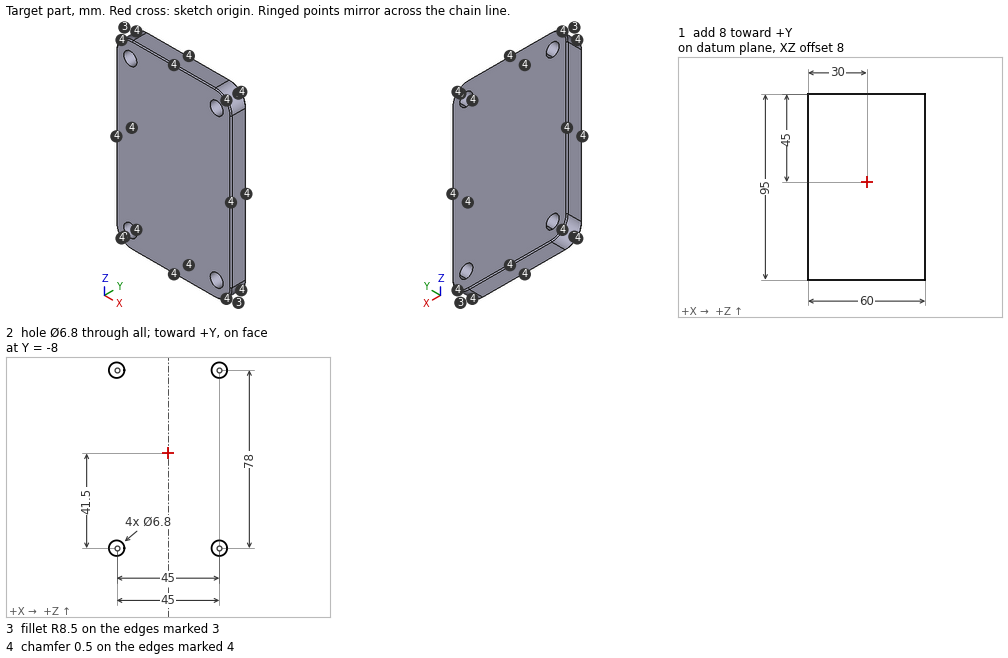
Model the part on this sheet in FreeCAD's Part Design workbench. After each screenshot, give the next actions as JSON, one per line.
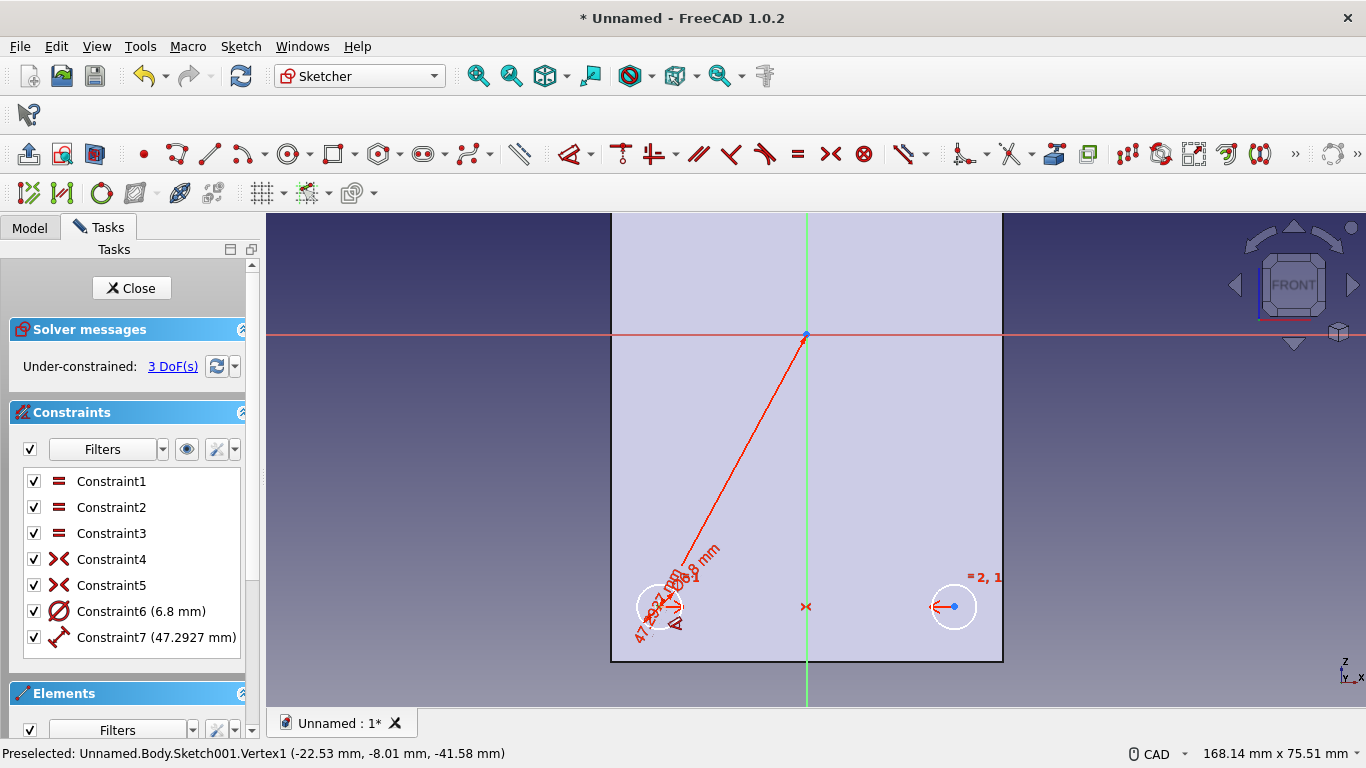
{"action": "left_click", "coordinate": [954, 607]}
{"action": "left_click", "coordinate": [739, 641]}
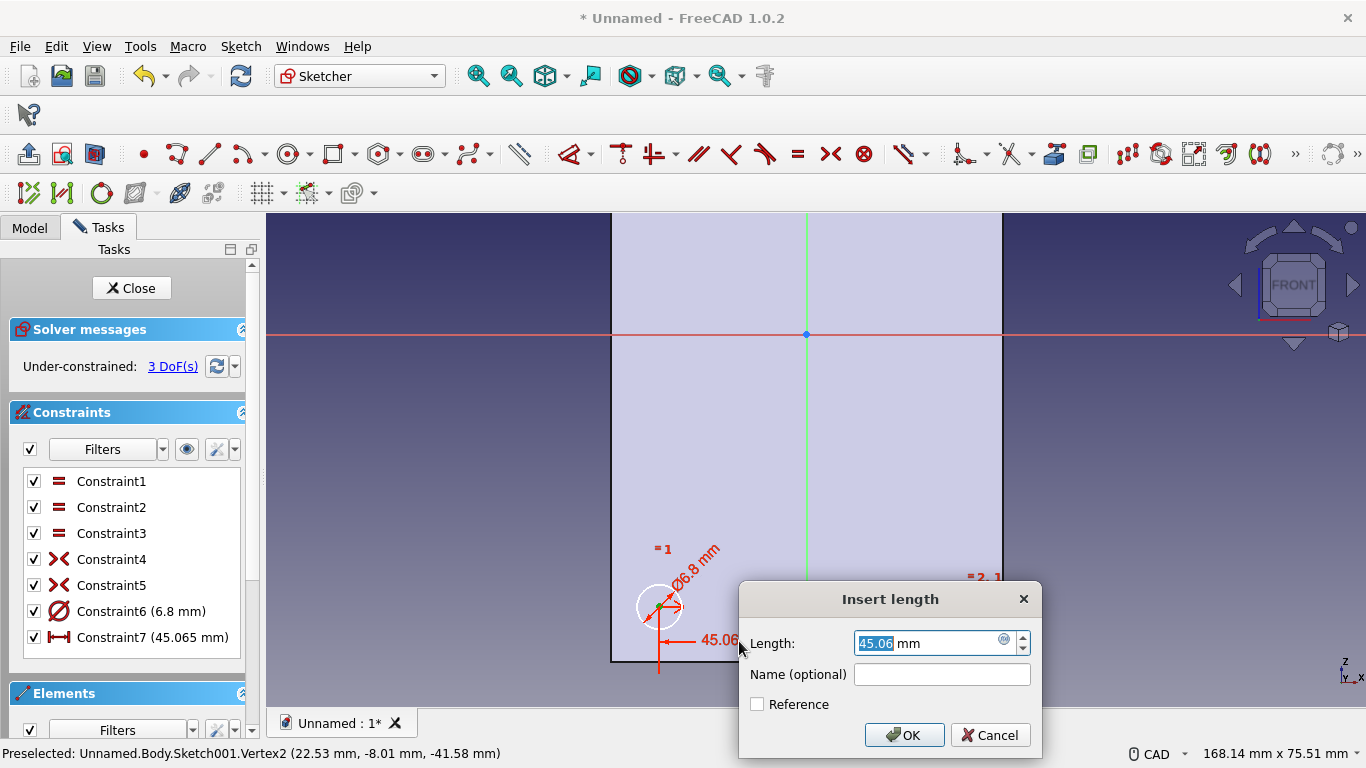
{"action": "type", "text": "45"}
{"action": "key", "text": "Return"}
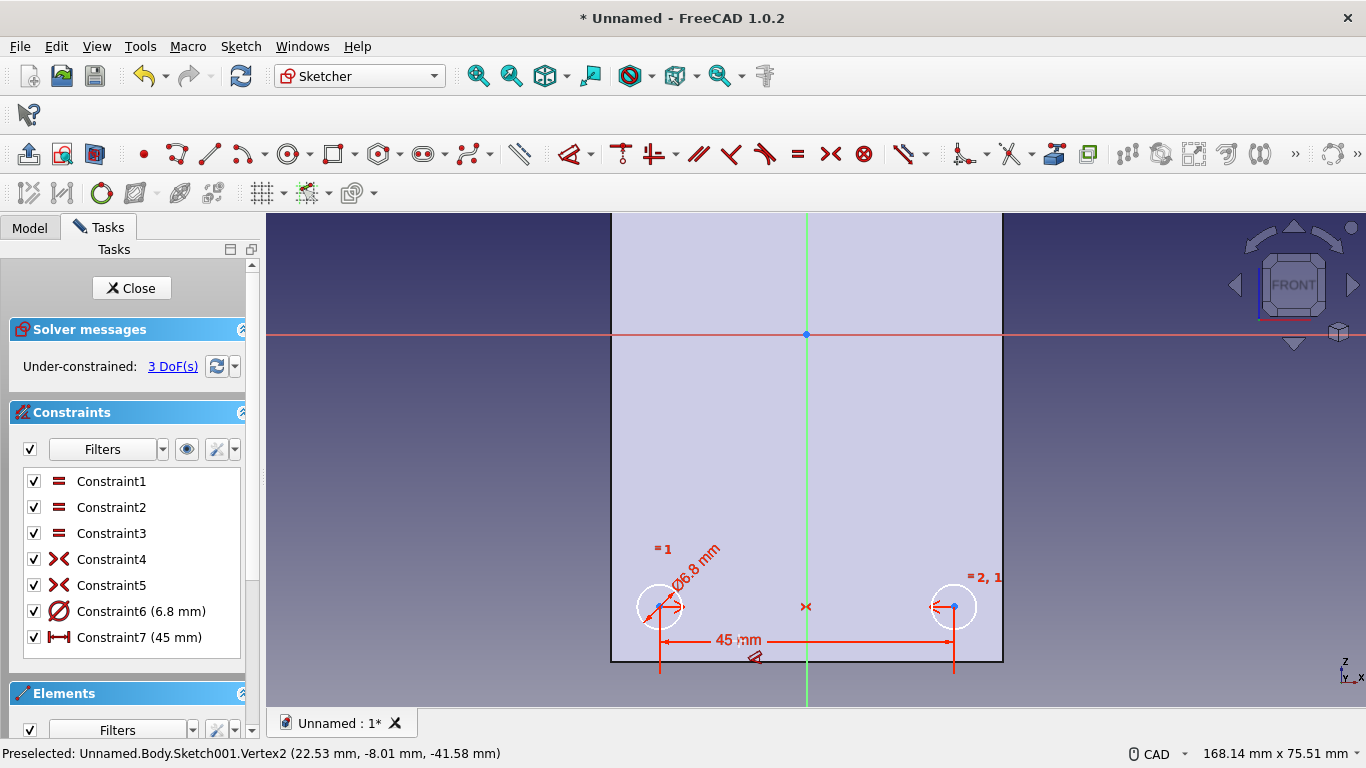
{"action": "left_click", "coordinate": [660, 607]}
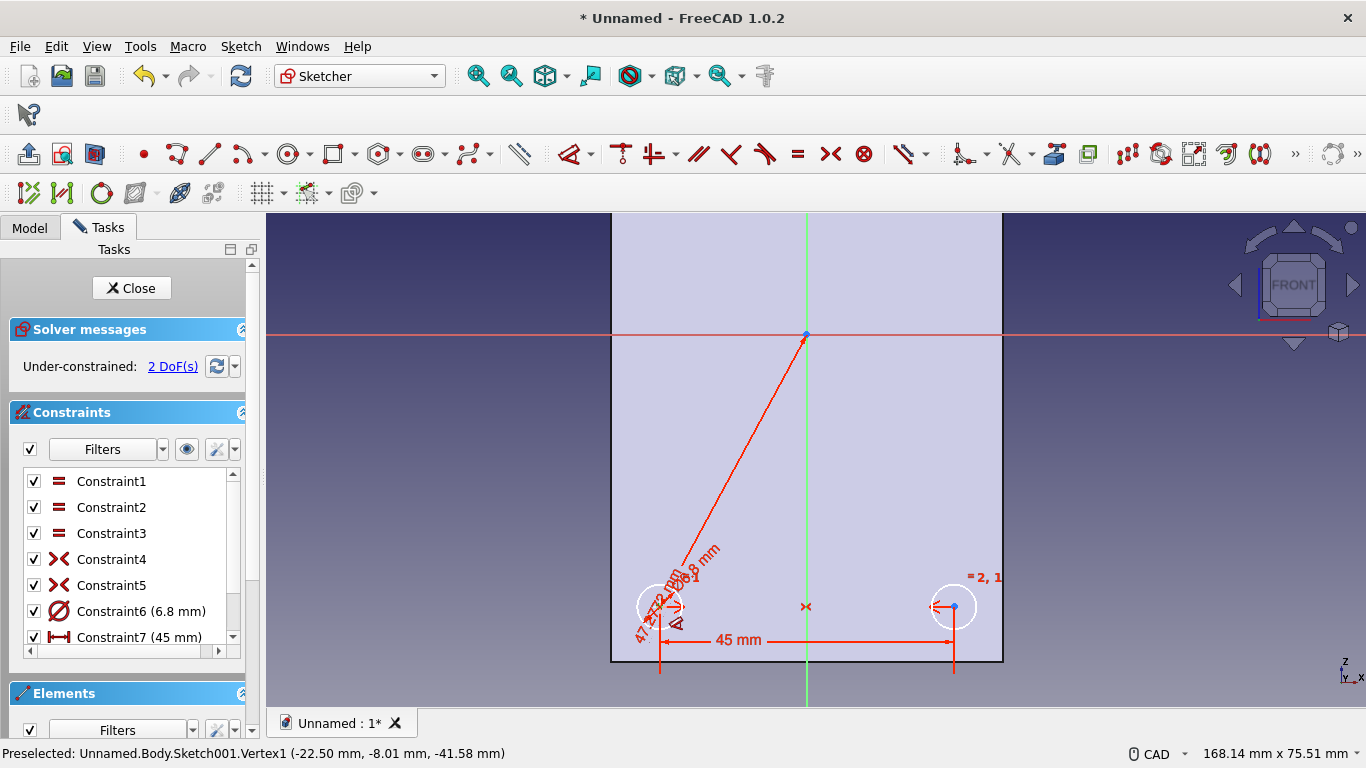
{"action": "scroll", "coordinate": [675, 592], "scroll_direction": "down", "scroll_amount": 3}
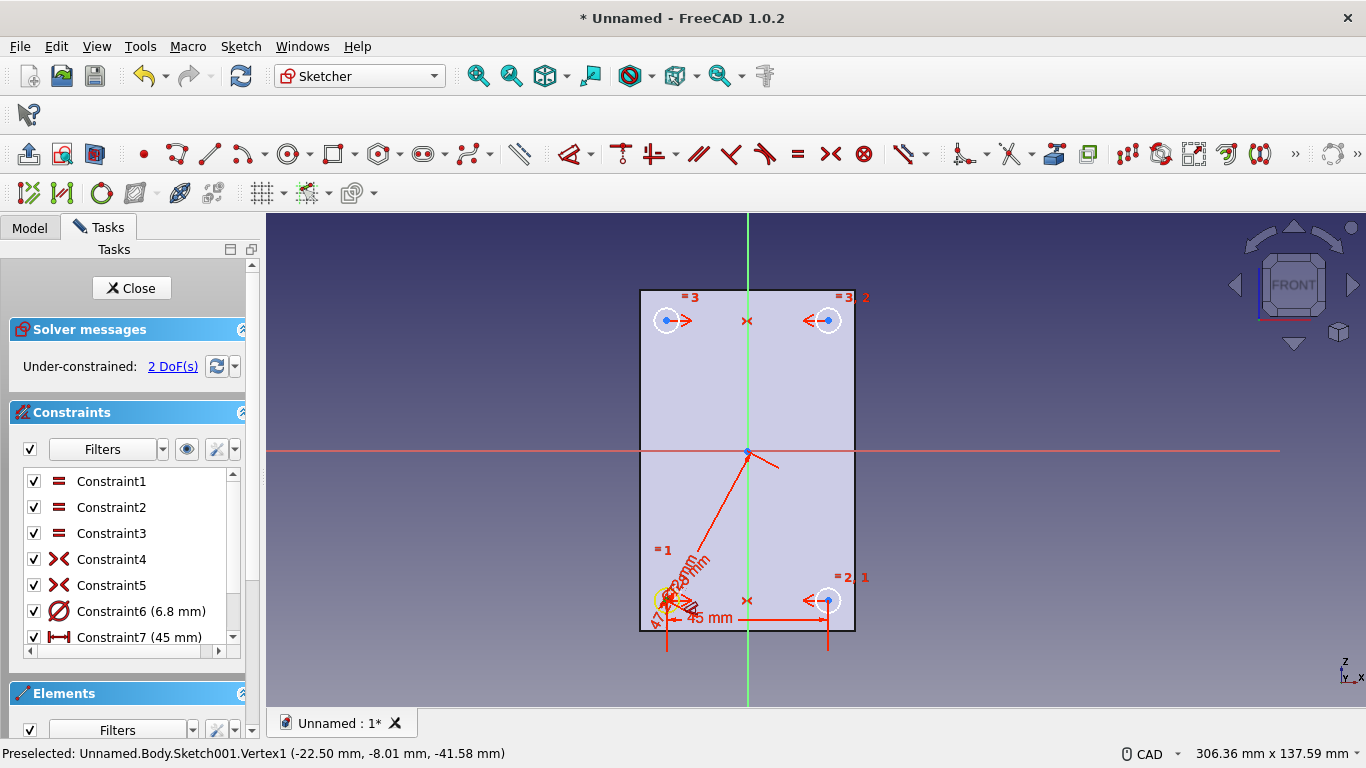
{"action": "left_click", "coordinate": [828, 321]}
{"action": "left_click", "coordinate": [785, 635]}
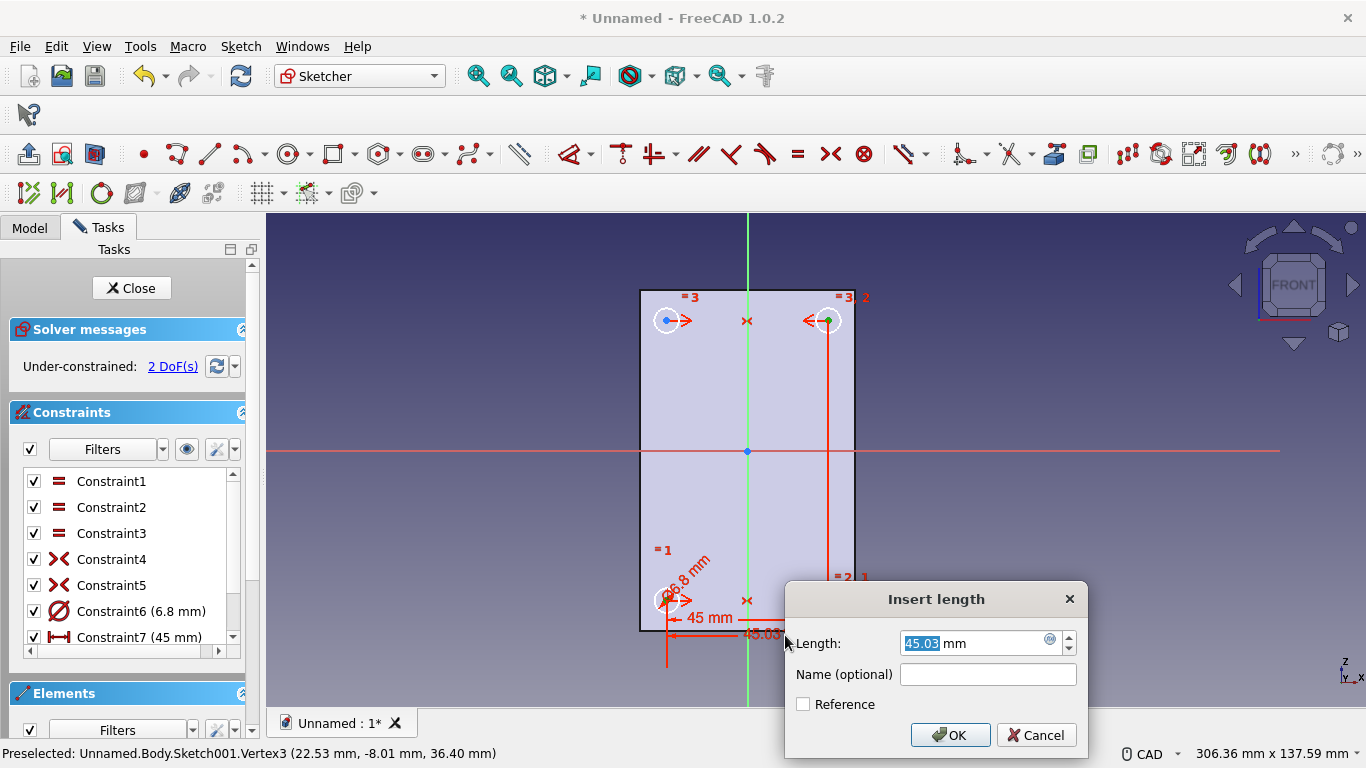
{"action": "type", "text": "45"}
{"action": "key", "text": "Return"}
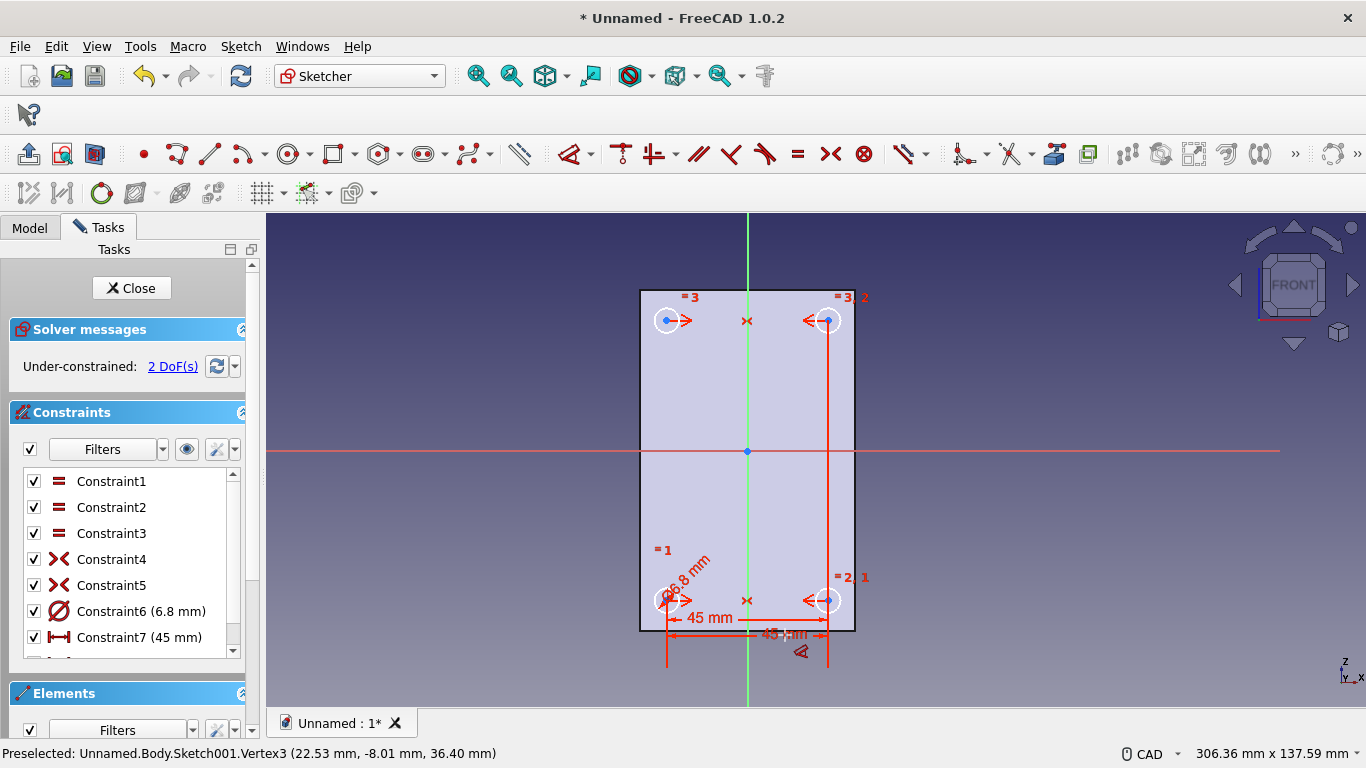
{"action": "left_click", "coordinate": [828, 601]}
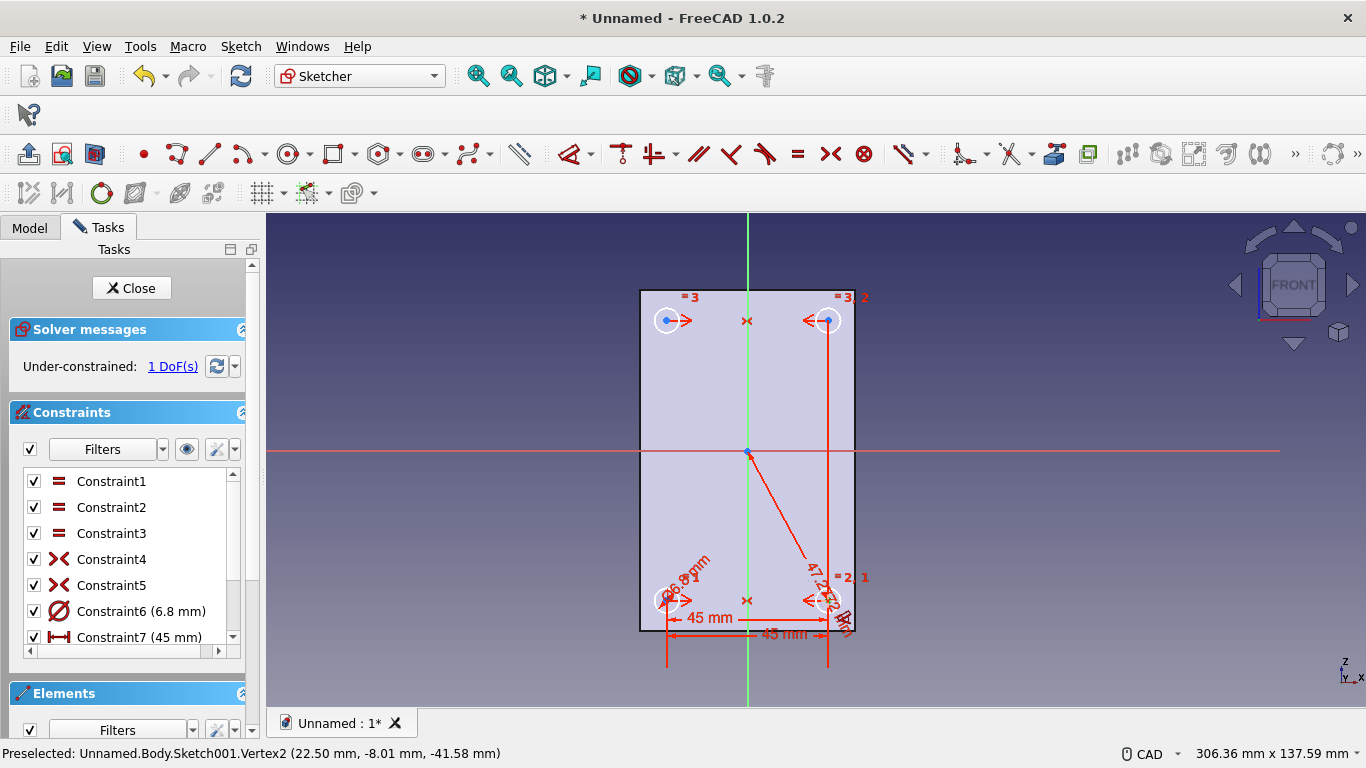
{"action": "left_click", "coordinate": [828, 321]}
{"action": "left_click", "coordinate": [862, 396]}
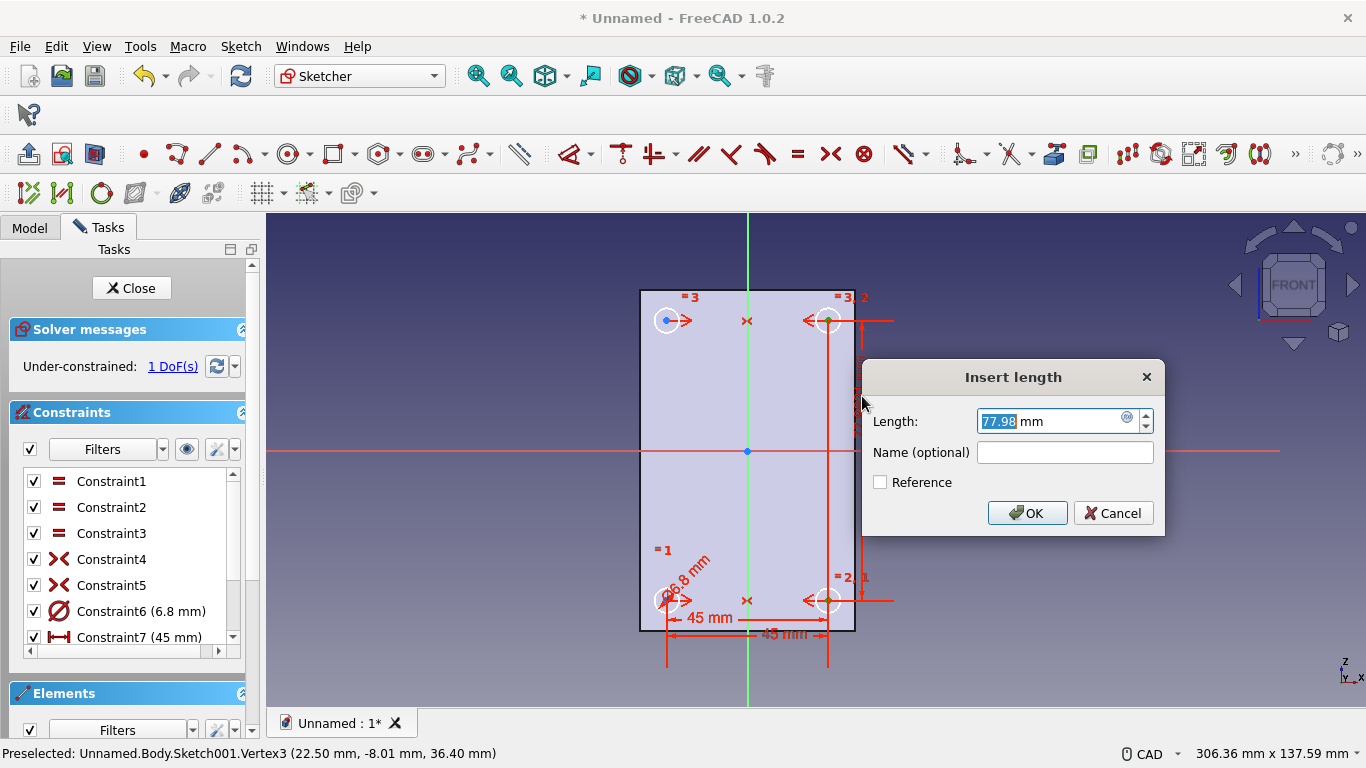
{"action": "type", "text": "78"}
{"action": "key", "text": "Return"}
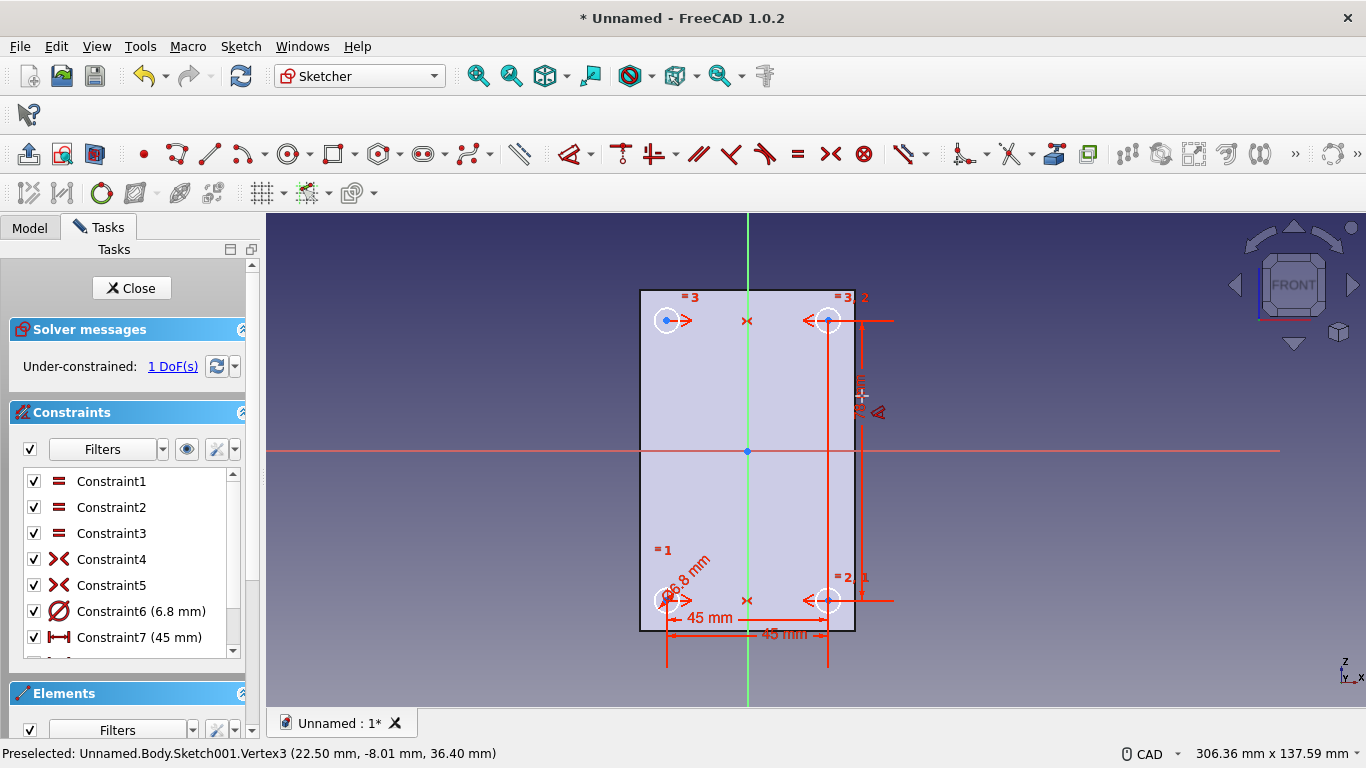
{"action": "left_click", "coordinate": [667, 601]}
{"action": "left_click", "coordinate": [633, 526]}